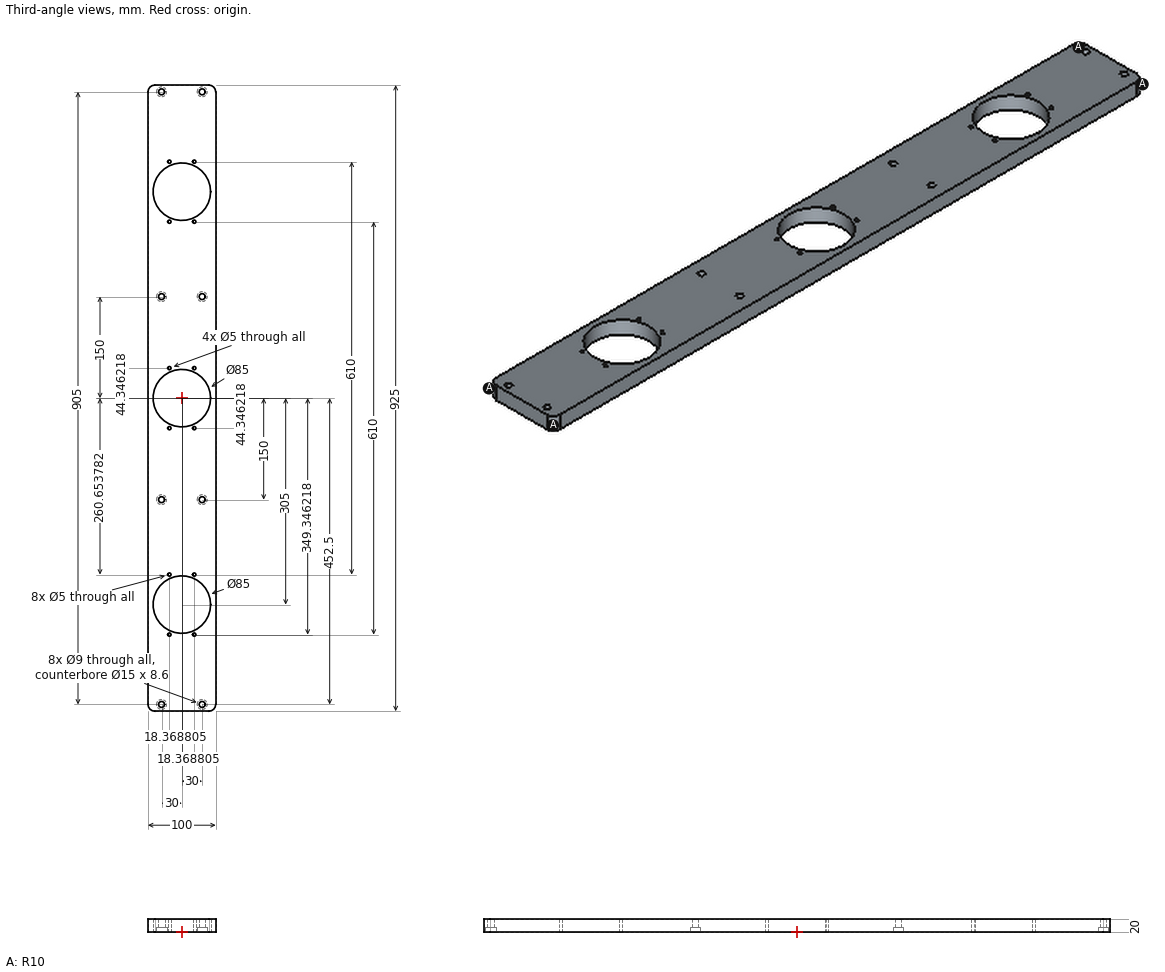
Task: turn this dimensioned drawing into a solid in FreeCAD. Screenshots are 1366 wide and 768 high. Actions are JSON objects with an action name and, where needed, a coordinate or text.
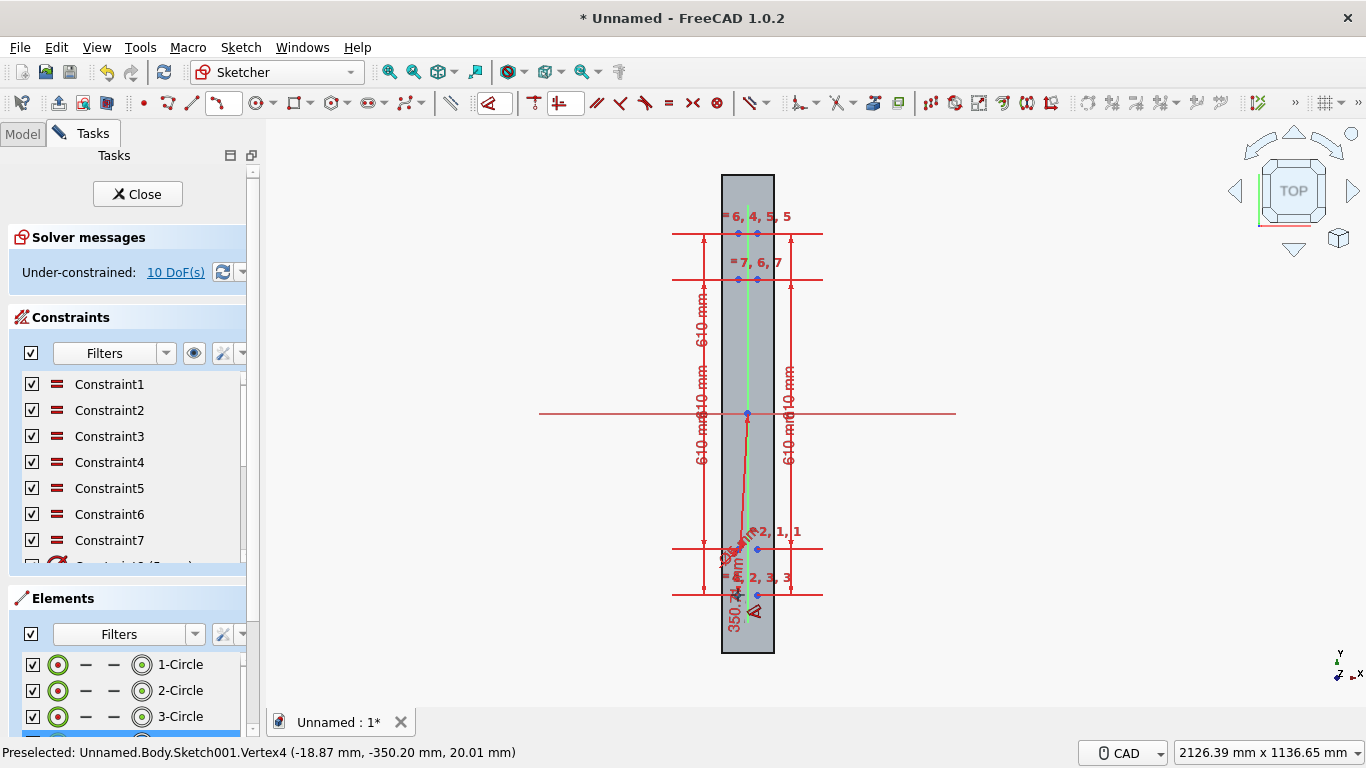
{"action": "left_click", "coordinate": [738, 280]}
{"action": "left_click", "coordinate": [704, 365]}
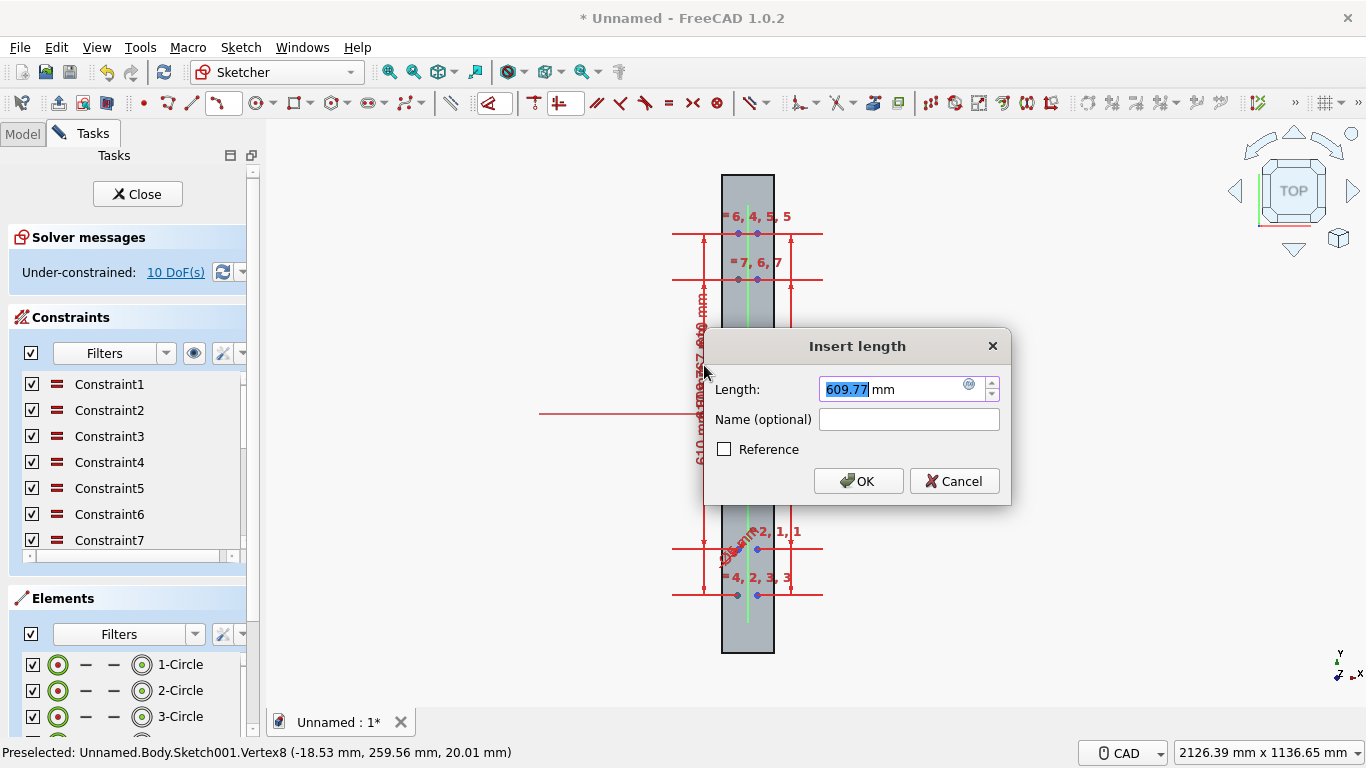
{"action": "type", "text": "610"}
{"action": "key", "text": "Return"}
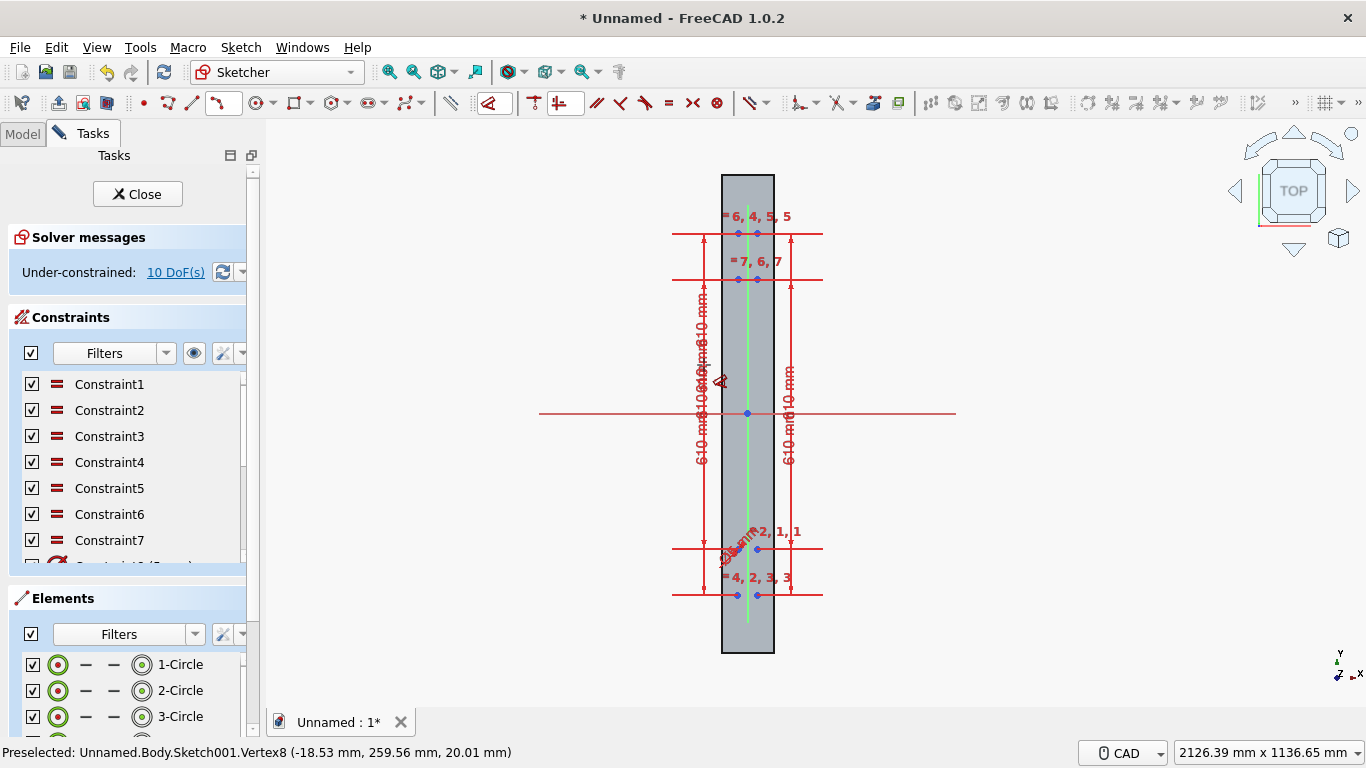
{"action": "scroll", "coordinate": [738, 549], "scroll_direction": "up", "scroll_amount": 8}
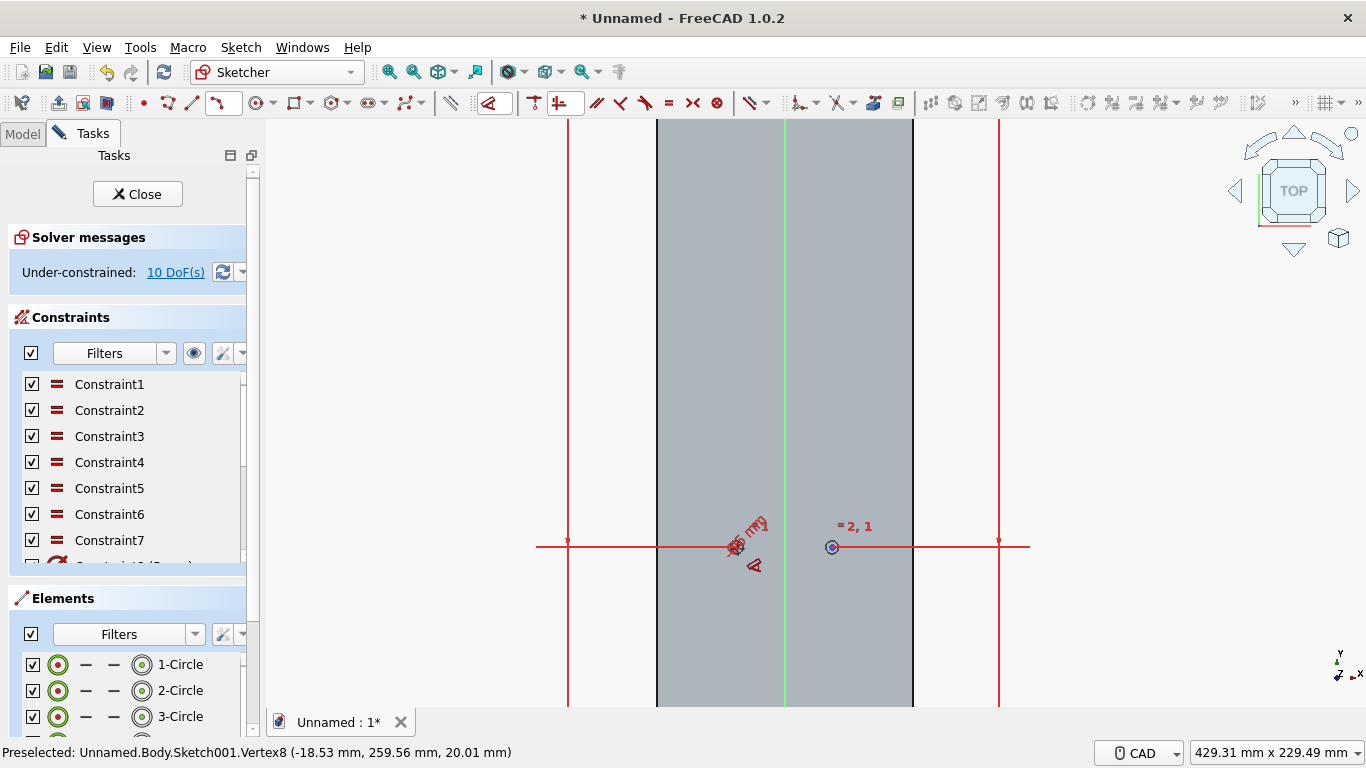
{"action": "left_click", "coordinate": [737, 547]}
{"action": "left_click", "coordinate": [761, 581]}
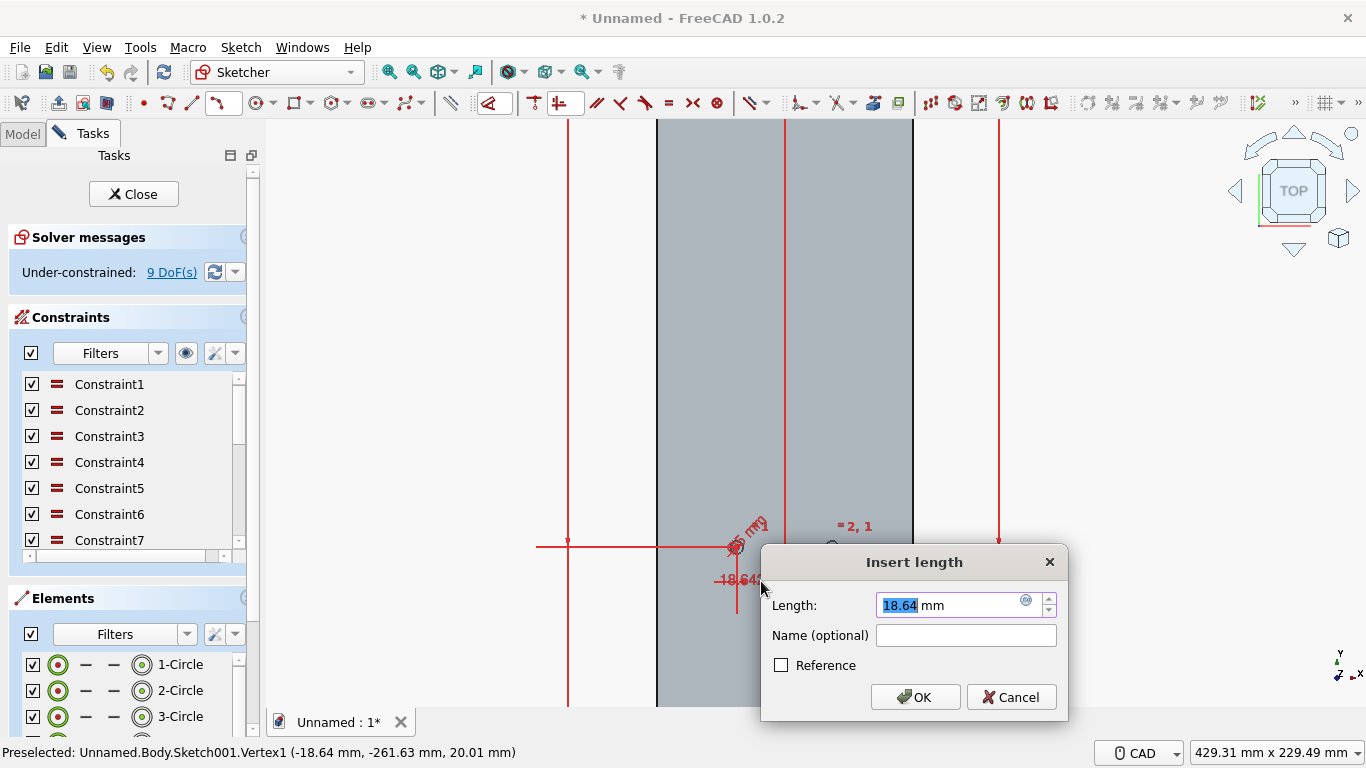
{"action": "type", "text": "18.368805"}
{"action": "key", "text": "Return"}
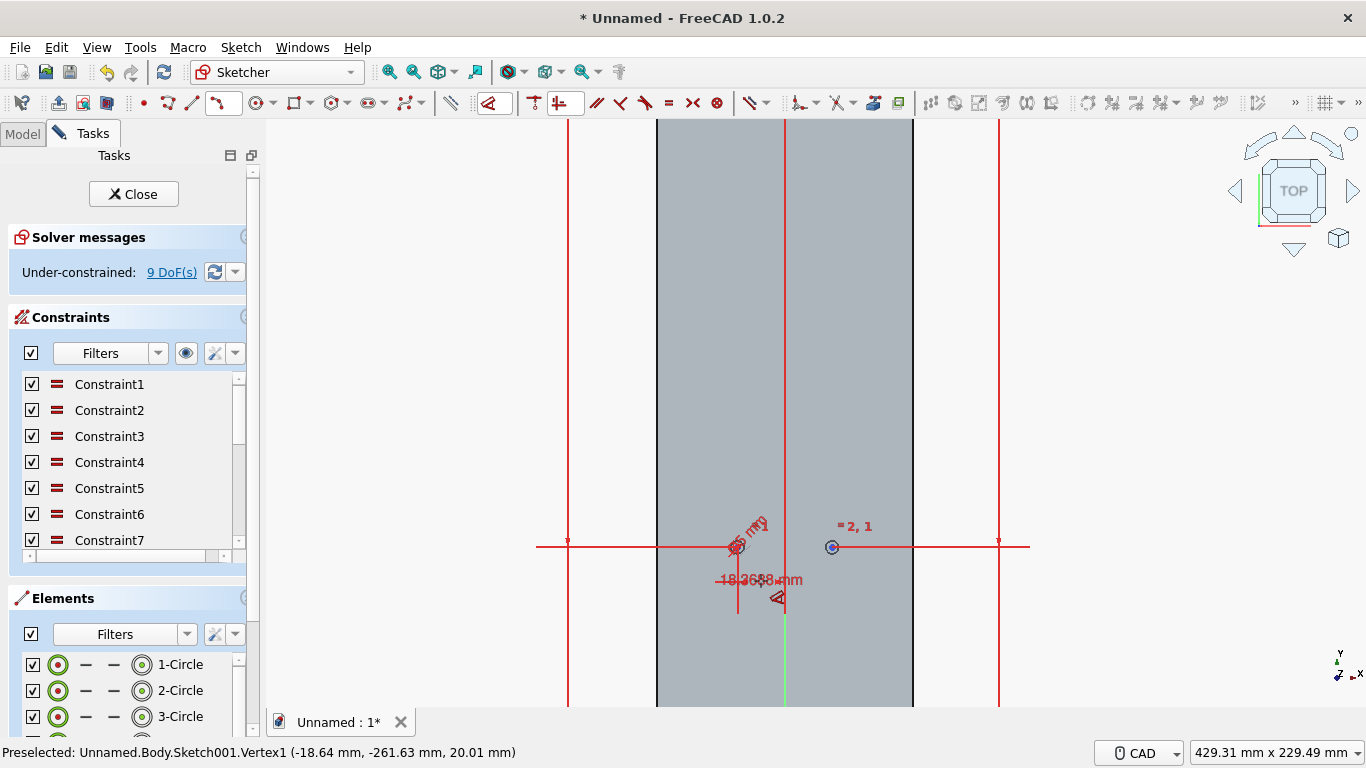
{"action": "left_click", "coordinate": [832, 547]}
{"action": "left_click", "coordinate": [808, 605]}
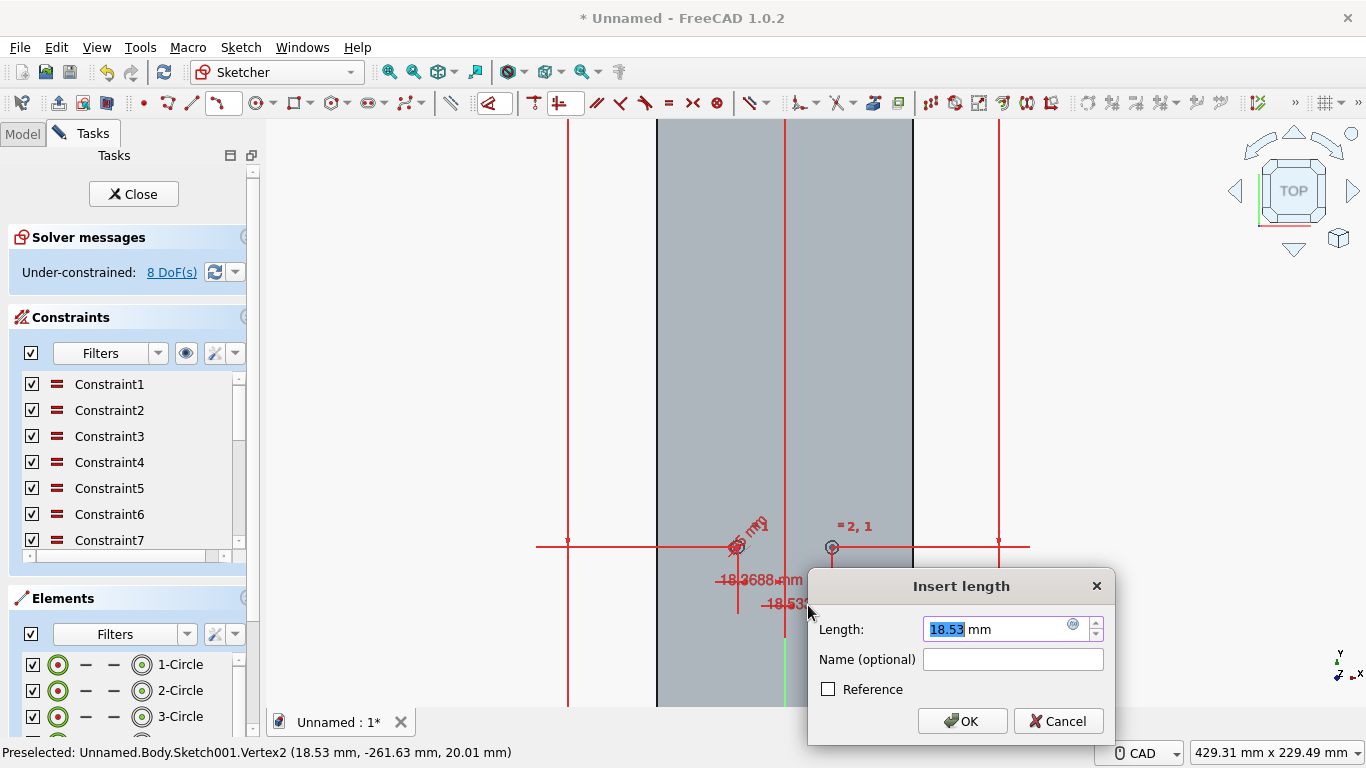
{"action": "type", "text": "18.368805"}
{"action": "key", "text": "Return"}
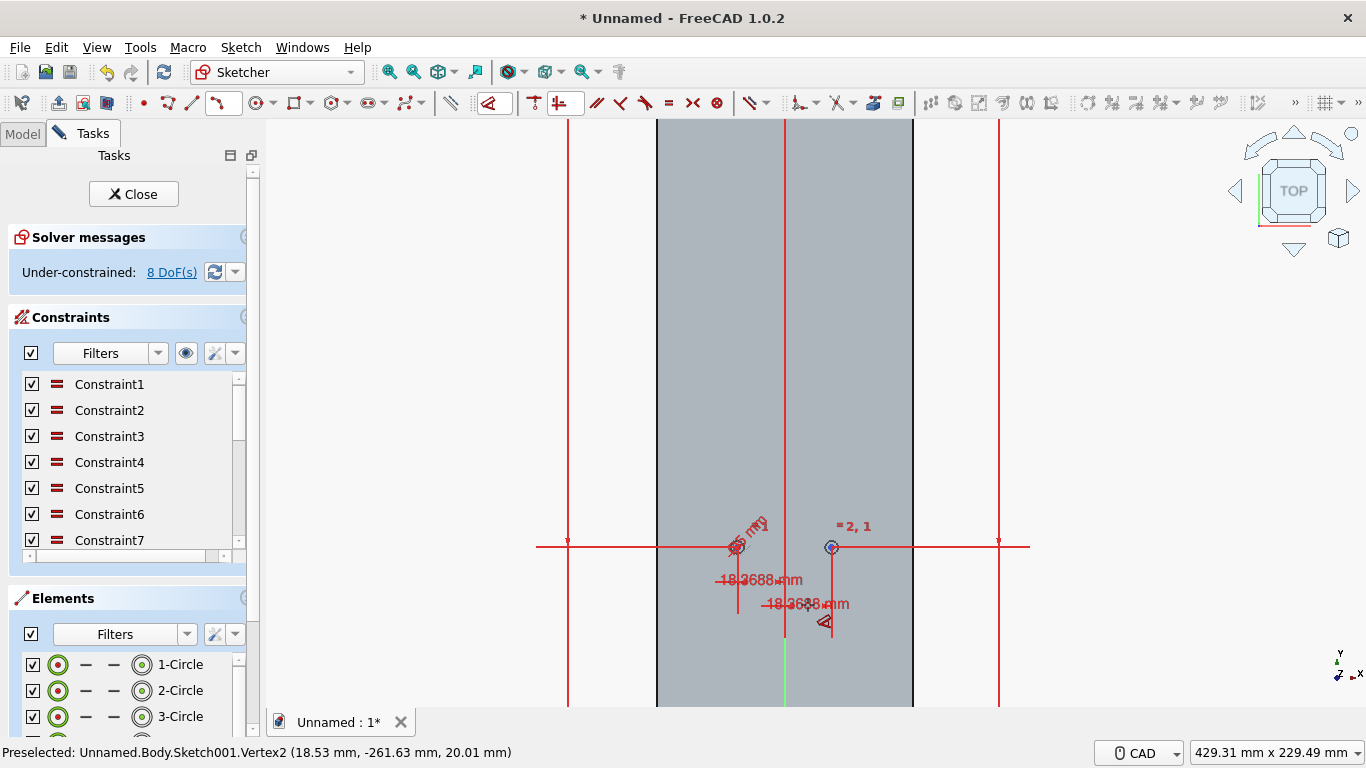
{"action": "scroll", "coordinate": [738, 549], "scroll_direction": "down", "scroll_amount": 8}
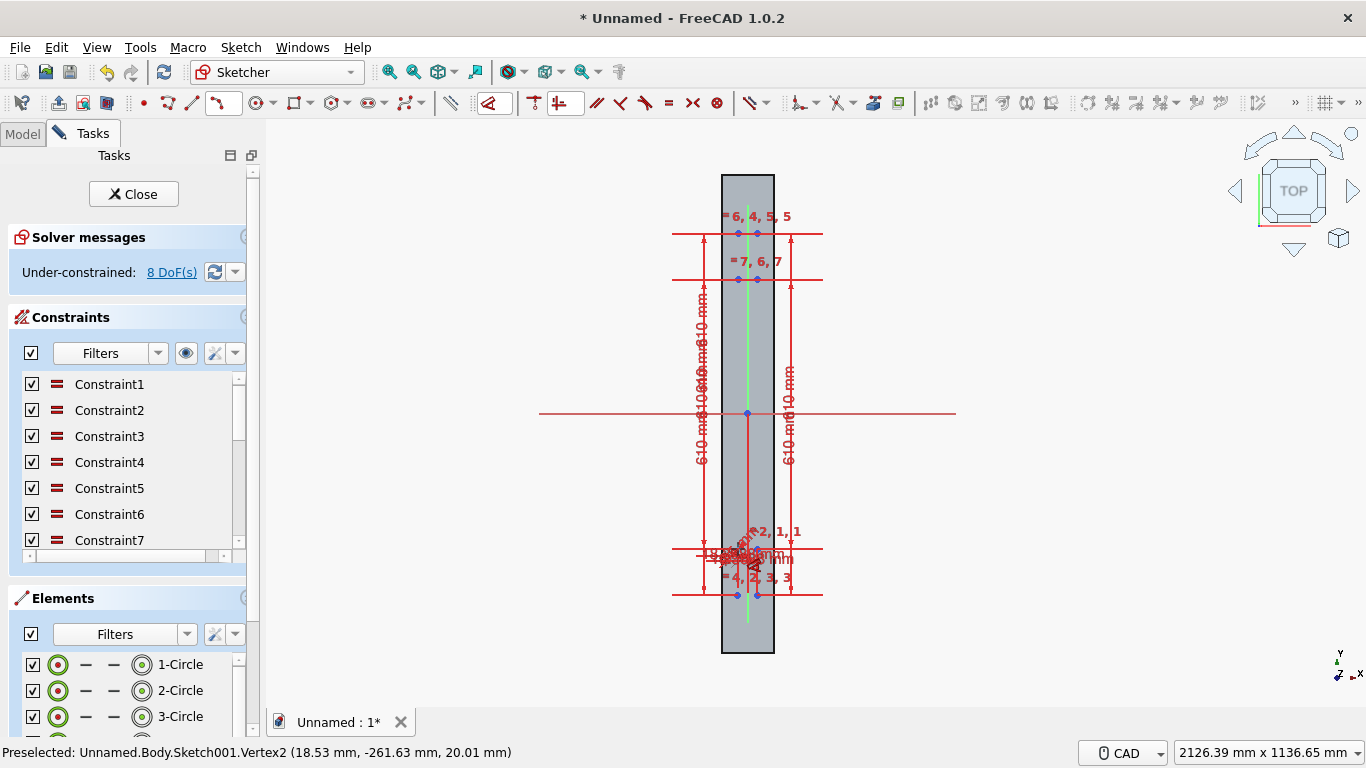
{"action": "scroll", "coordinate": [757, 595], "scroll_direction": "up", "scroll_amount": 8}